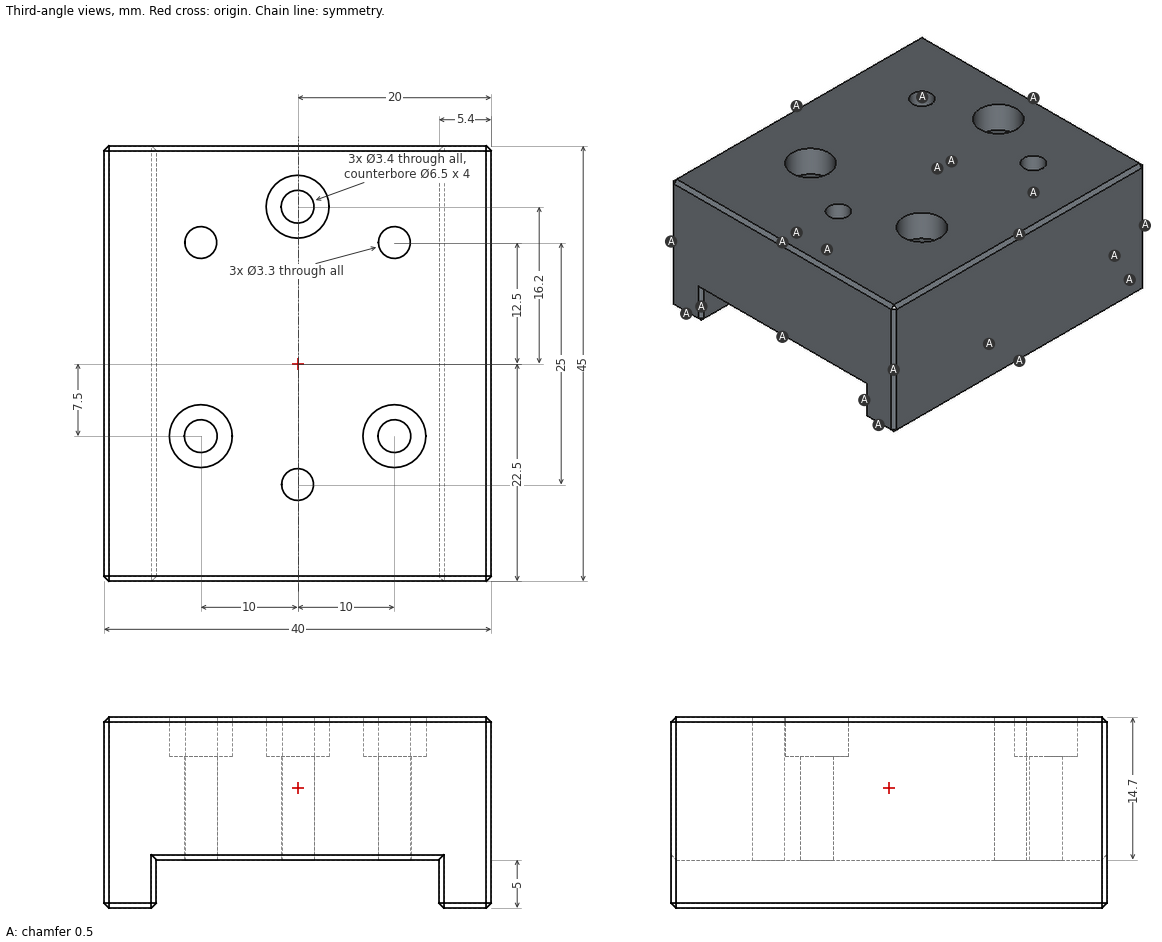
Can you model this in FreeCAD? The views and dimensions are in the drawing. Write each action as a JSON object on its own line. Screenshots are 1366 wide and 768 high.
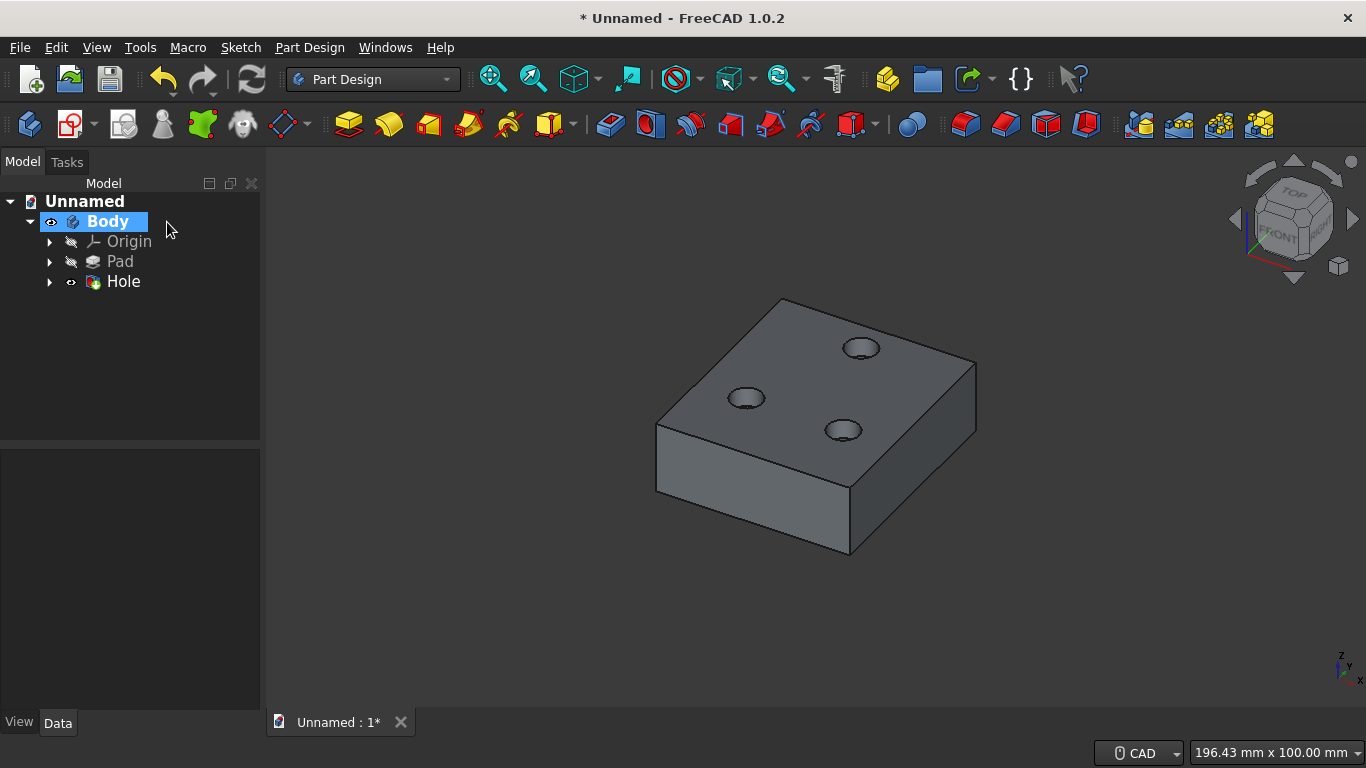
{"action": "key", "text": "5"}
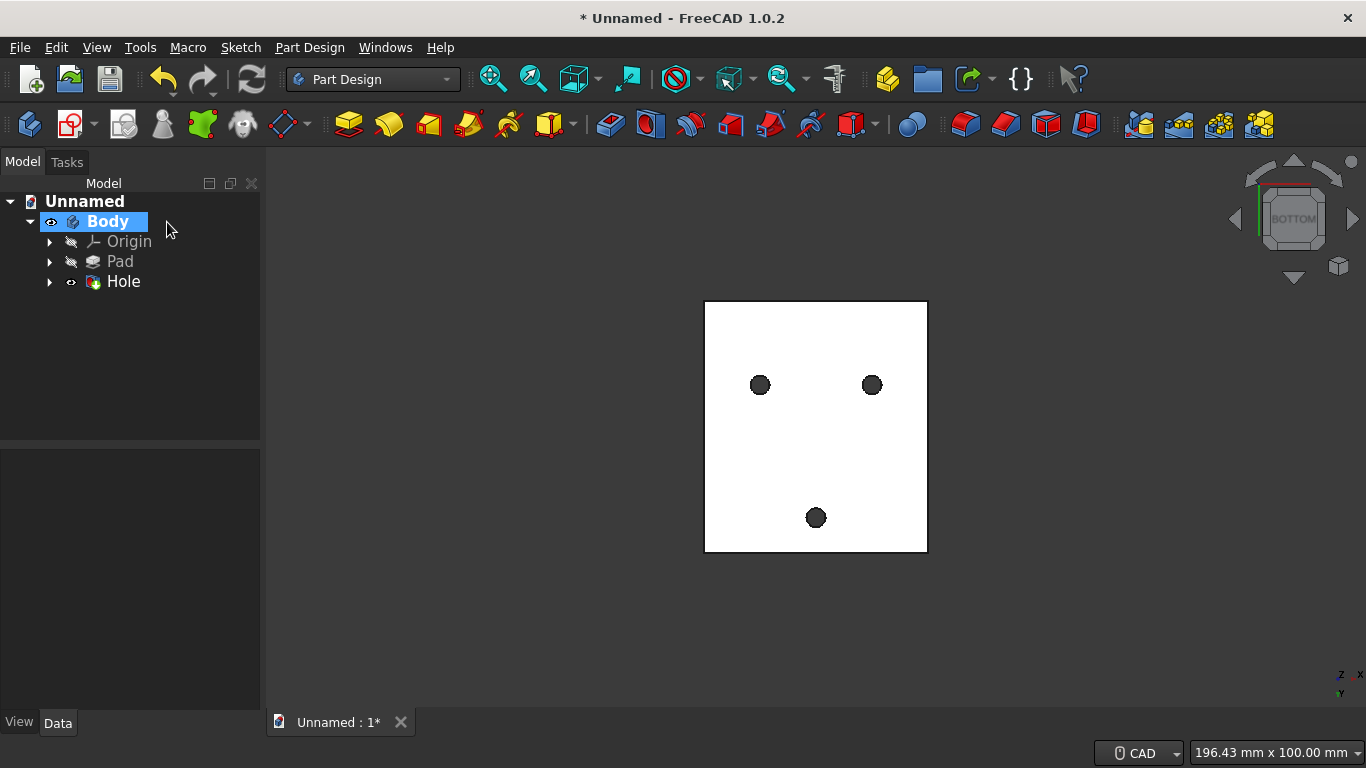
{"action": "left_click", "coordinate": [816, 426]}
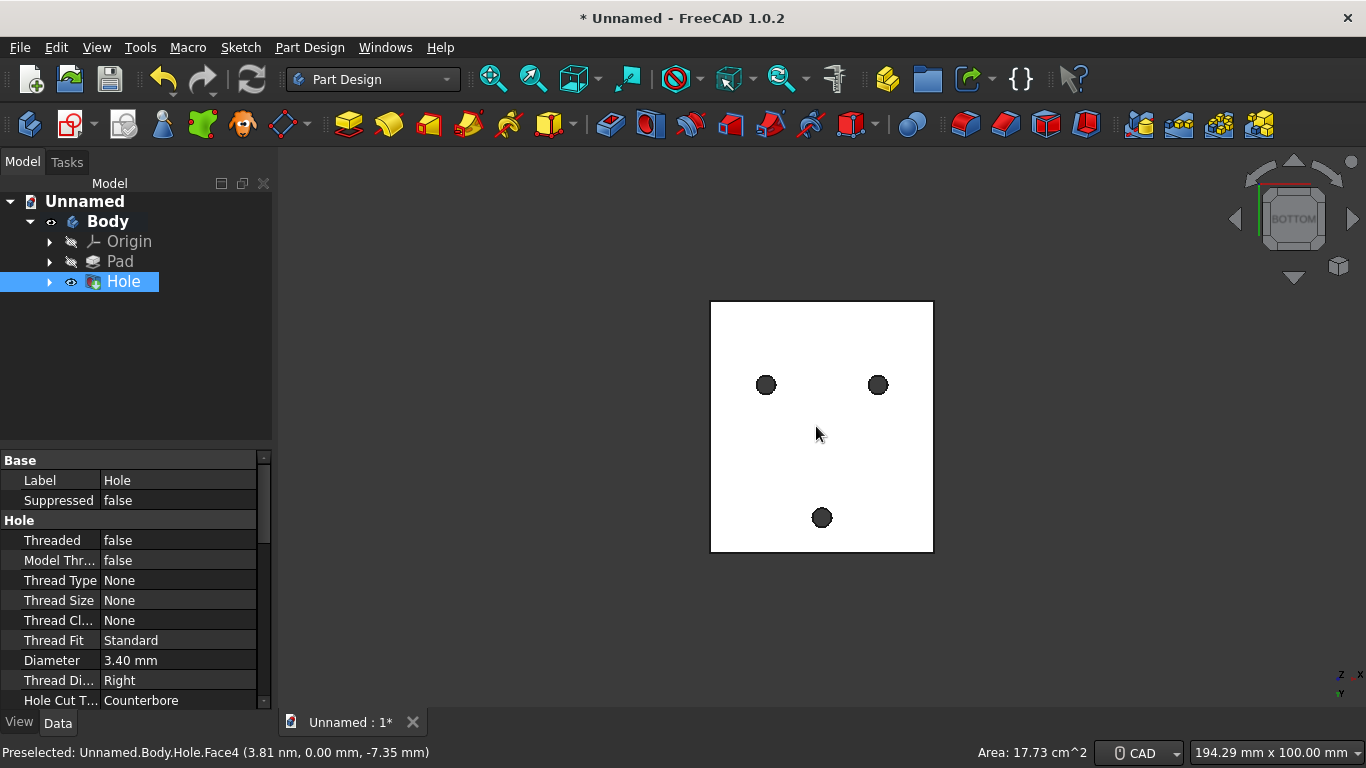
{"action": "left_click", "coordinate": [70, 124]}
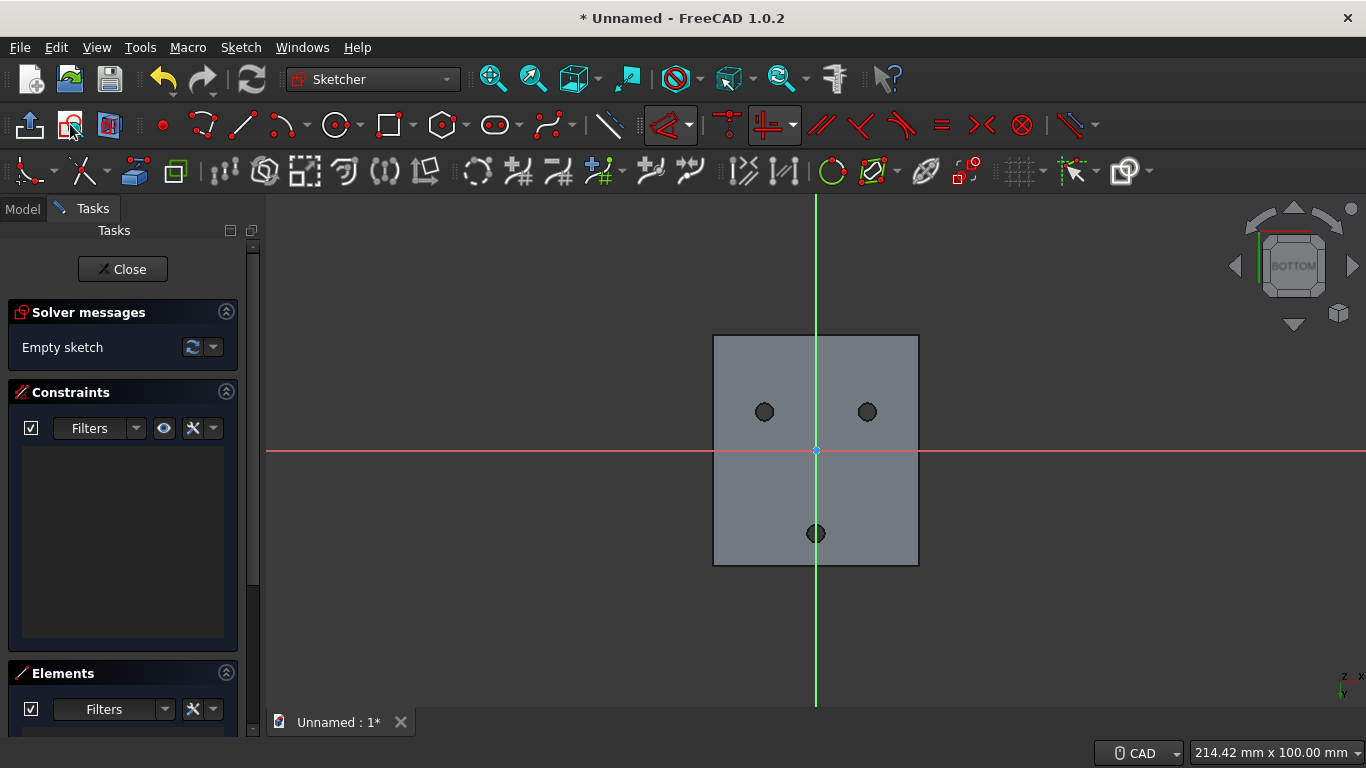
{"action": "scroll", "coordinate": [955, 451], "scroll_direction": "up", "scroll_amount": 2}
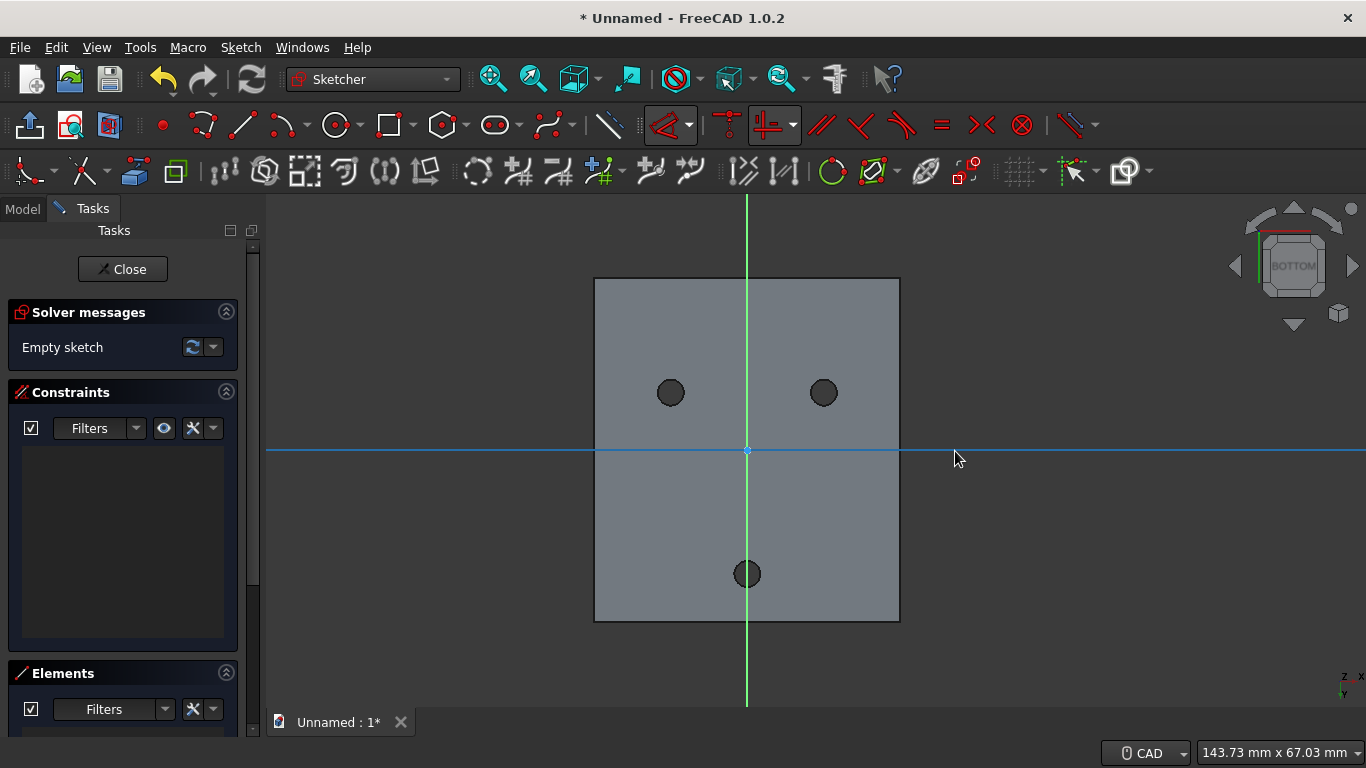
{"action": "left_click", "coordinate": [390, 126]}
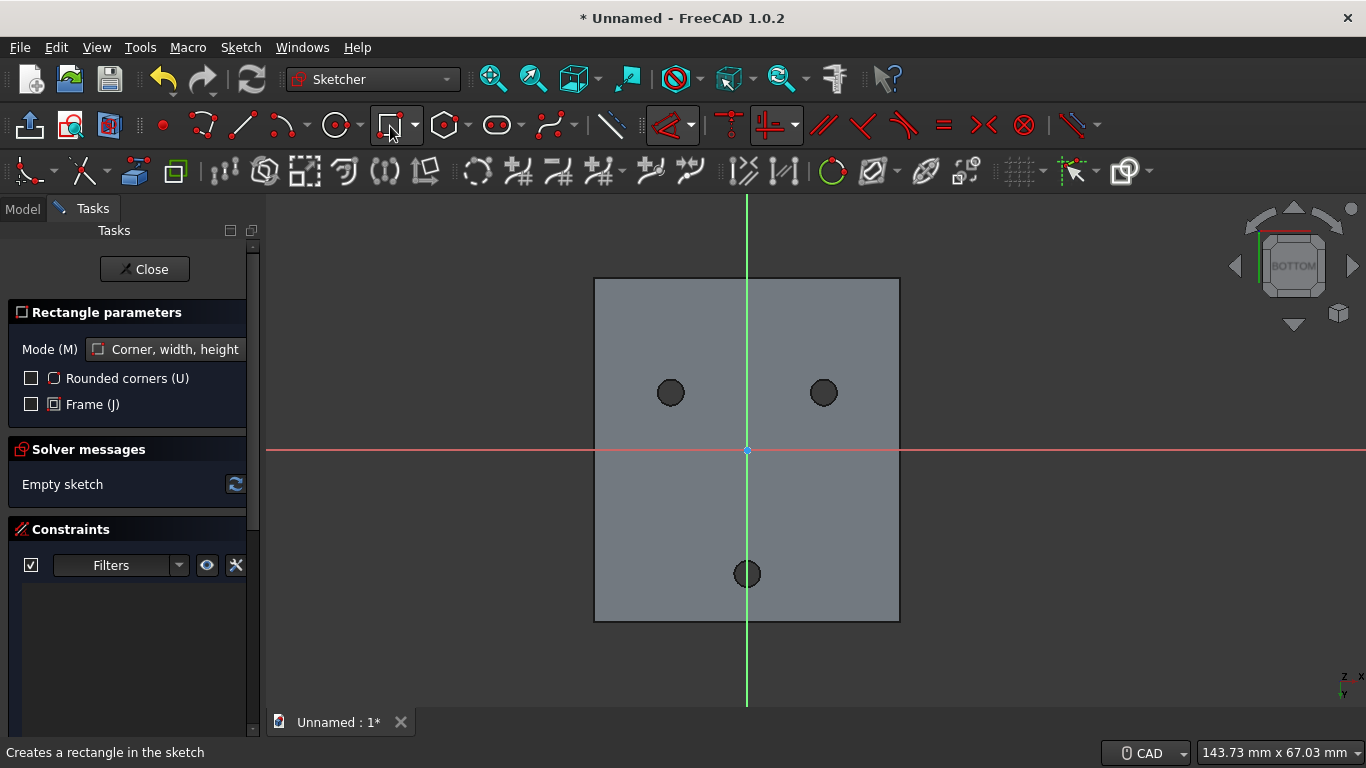
{"action": "left_click", "coordinate": [859, 278]}
{"action": "left_click", "coordinate": [900, 622]}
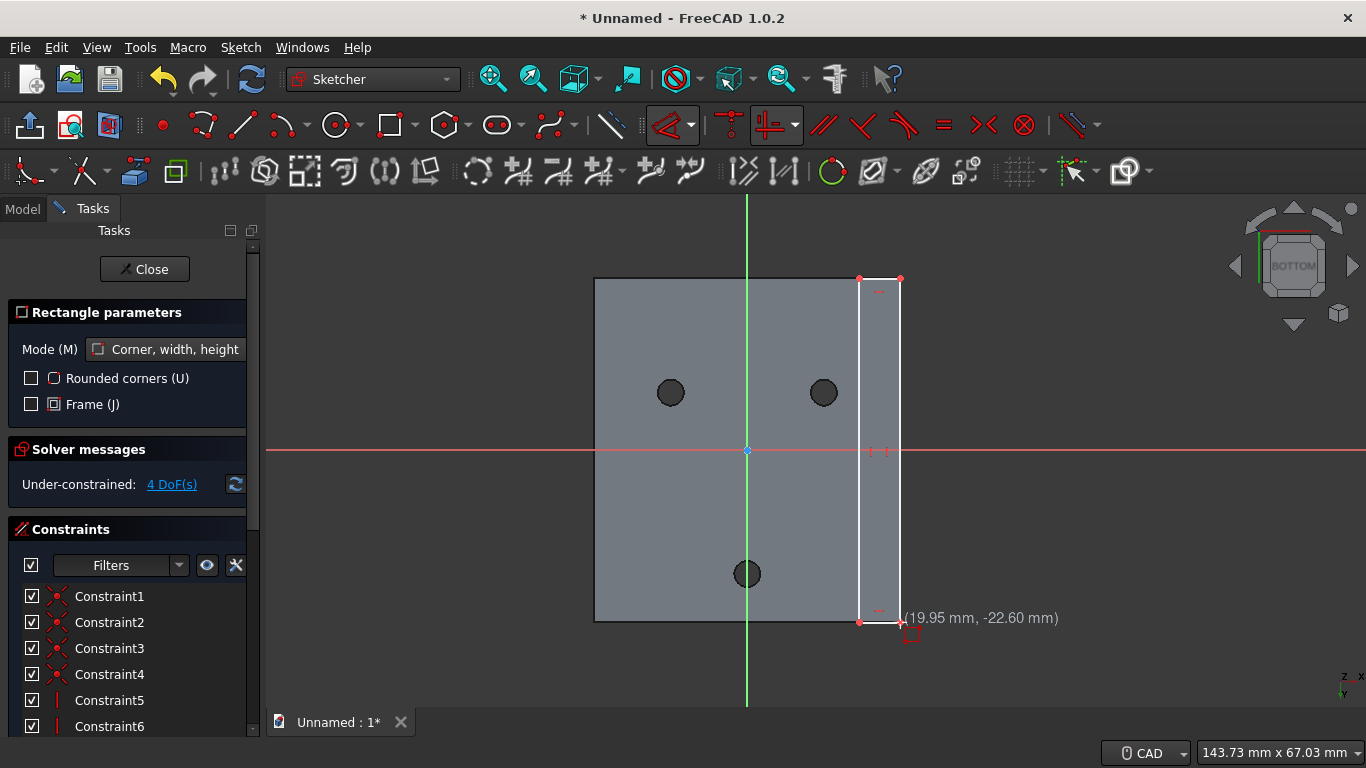
{"action": "left_click", "coordinate": [594, 278]}
{"action": "left_click", "coordinate": [636, 622]}
{"action": "key", "text": "Escape"}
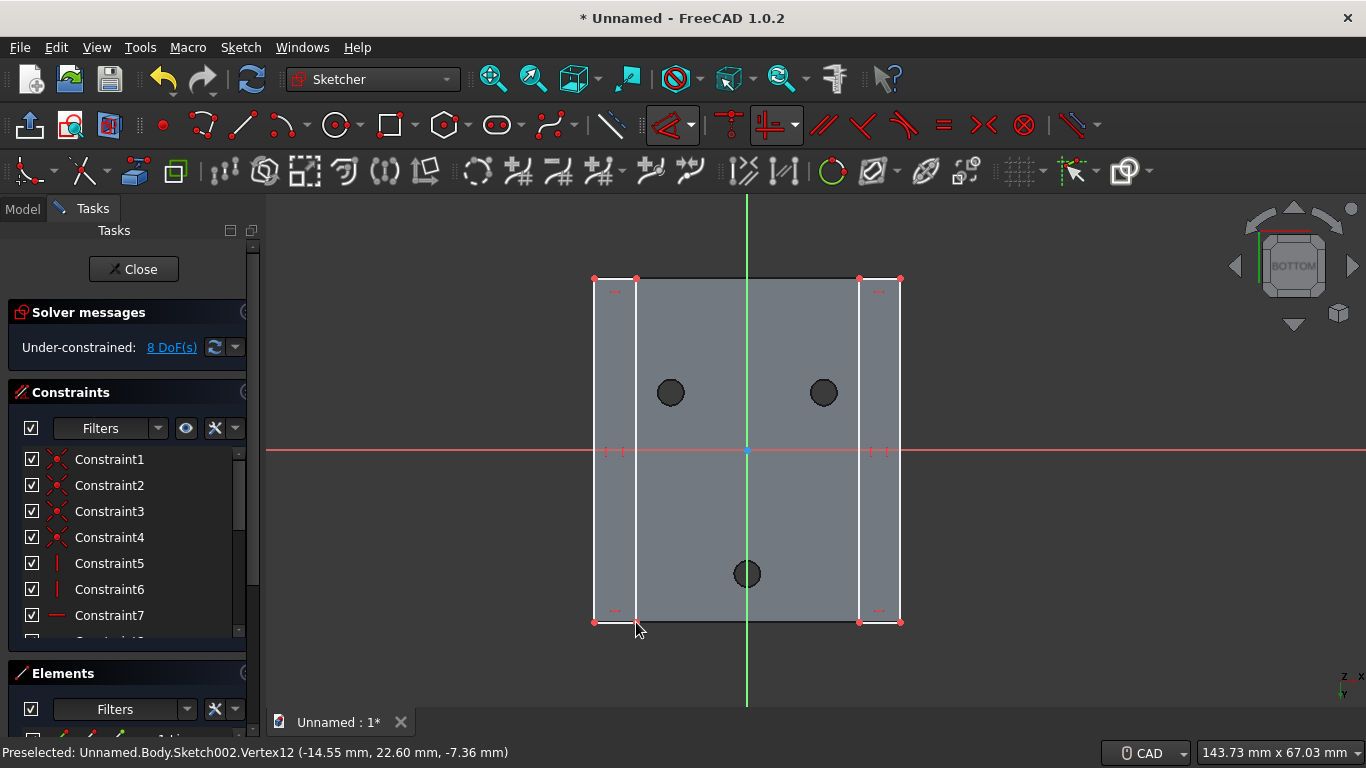
{"action": "left_click", "coordinate": [900, 279]}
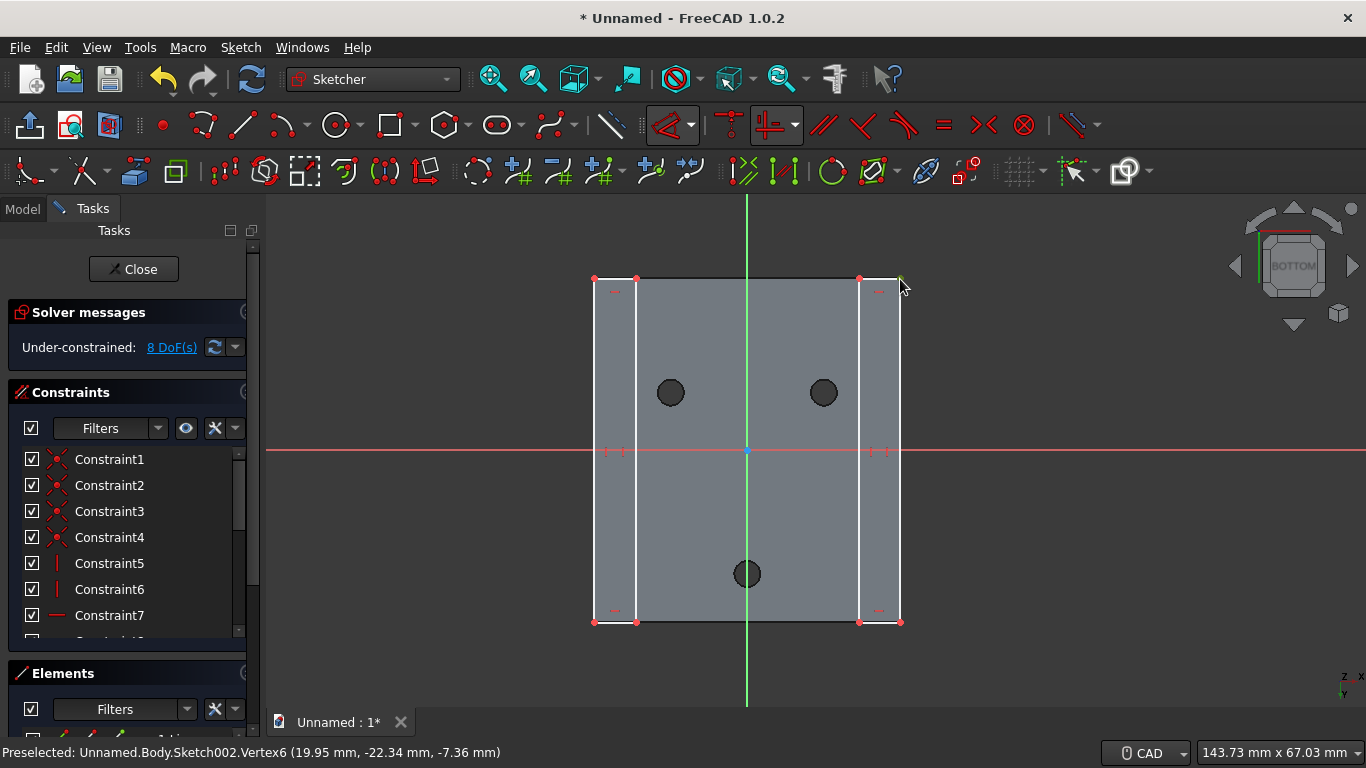
{"action": "left_click", "coordinate": [594, 279]}